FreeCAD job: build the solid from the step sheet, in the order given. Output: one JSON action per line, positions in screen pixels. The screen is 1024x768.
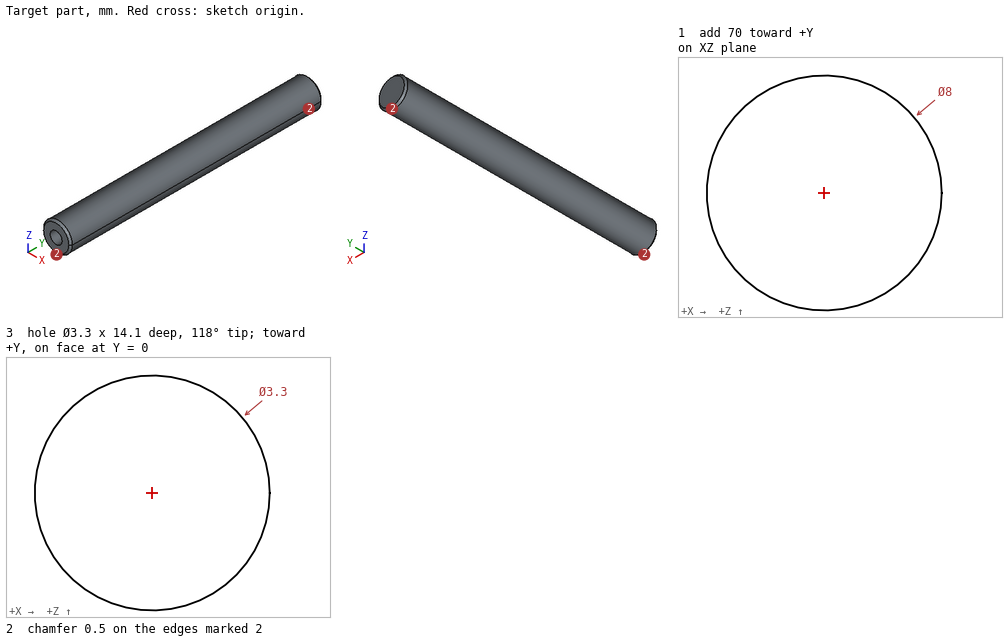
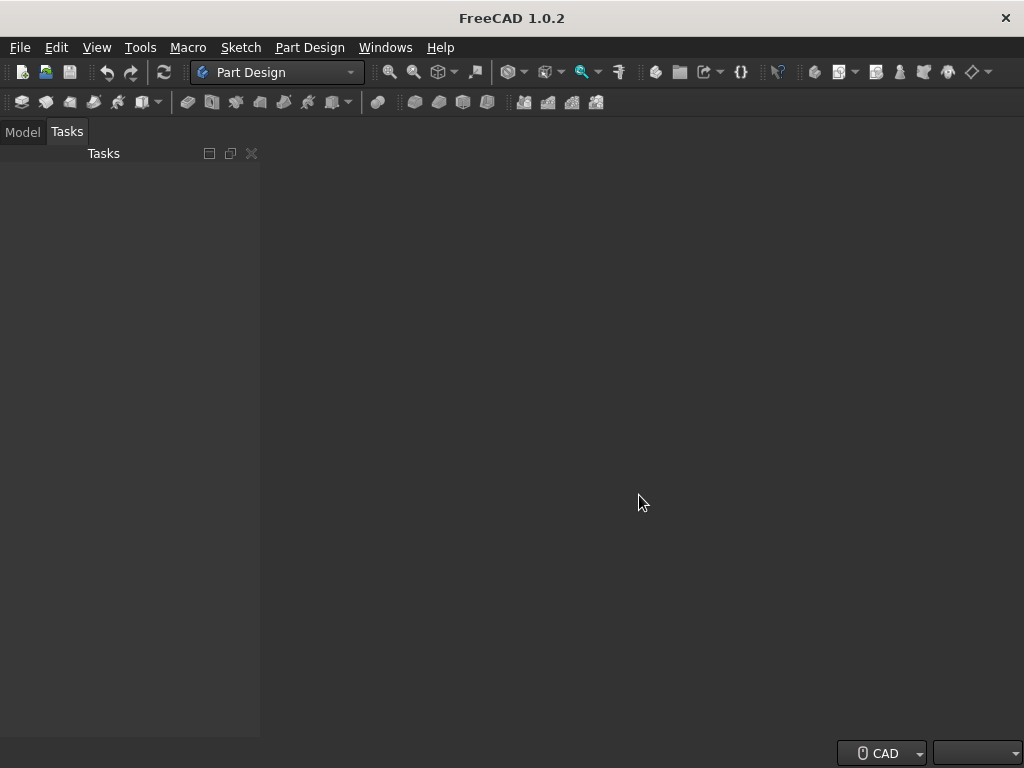
{"action": "key", "text": "ctrl+n"}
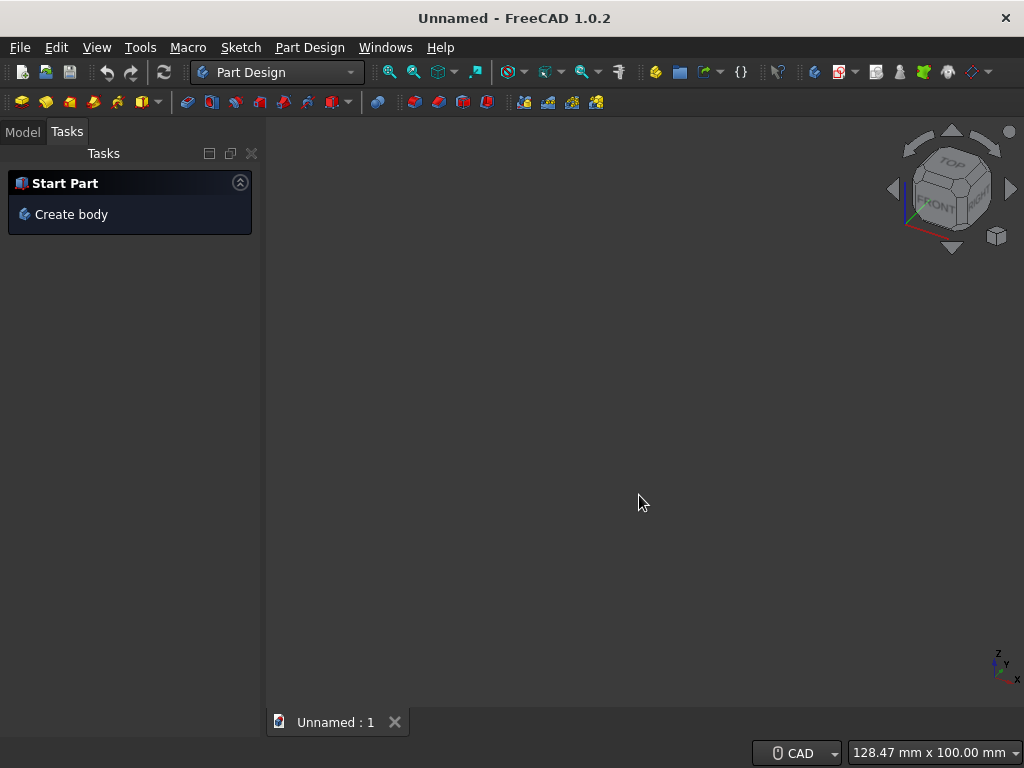
{"action": "left_click", "coordinate": [840, 72]}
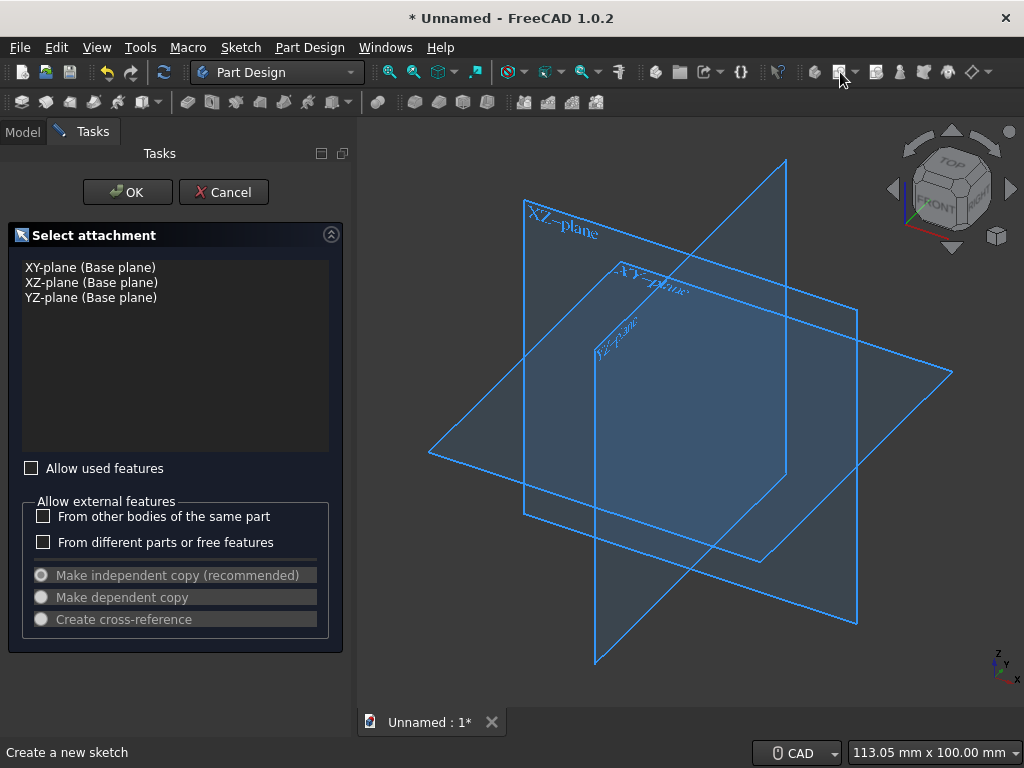
{"action": "left_click", "coordinate": [82, 282]}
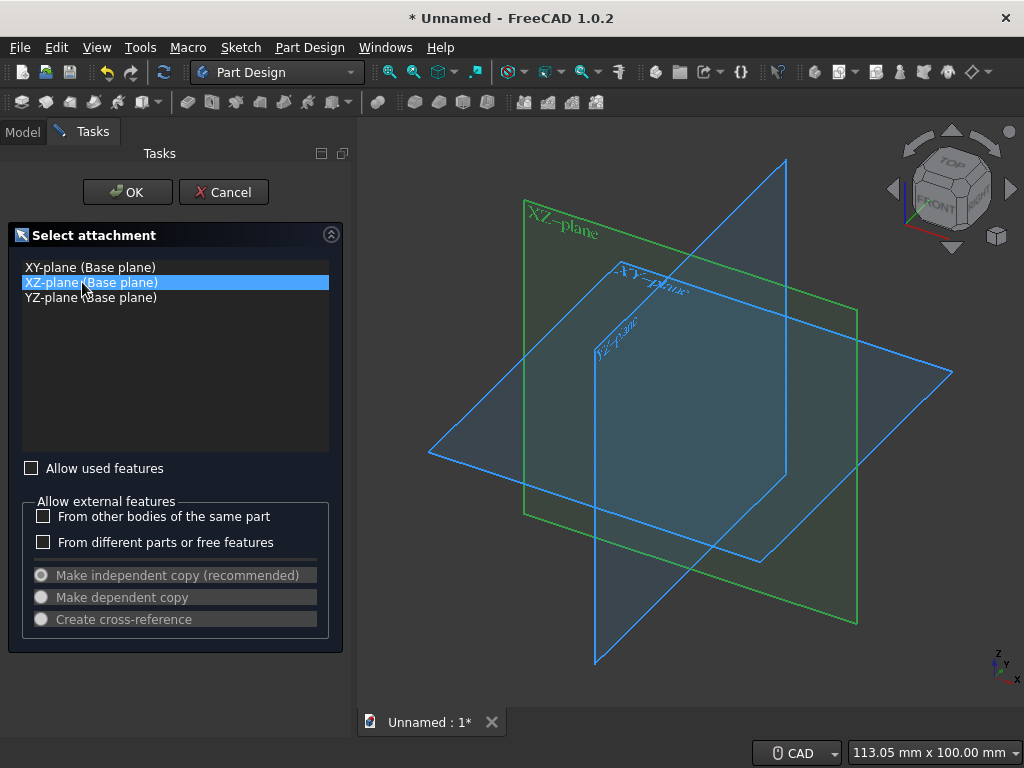
{"action": "left_click", "coordinate": [128, 192]}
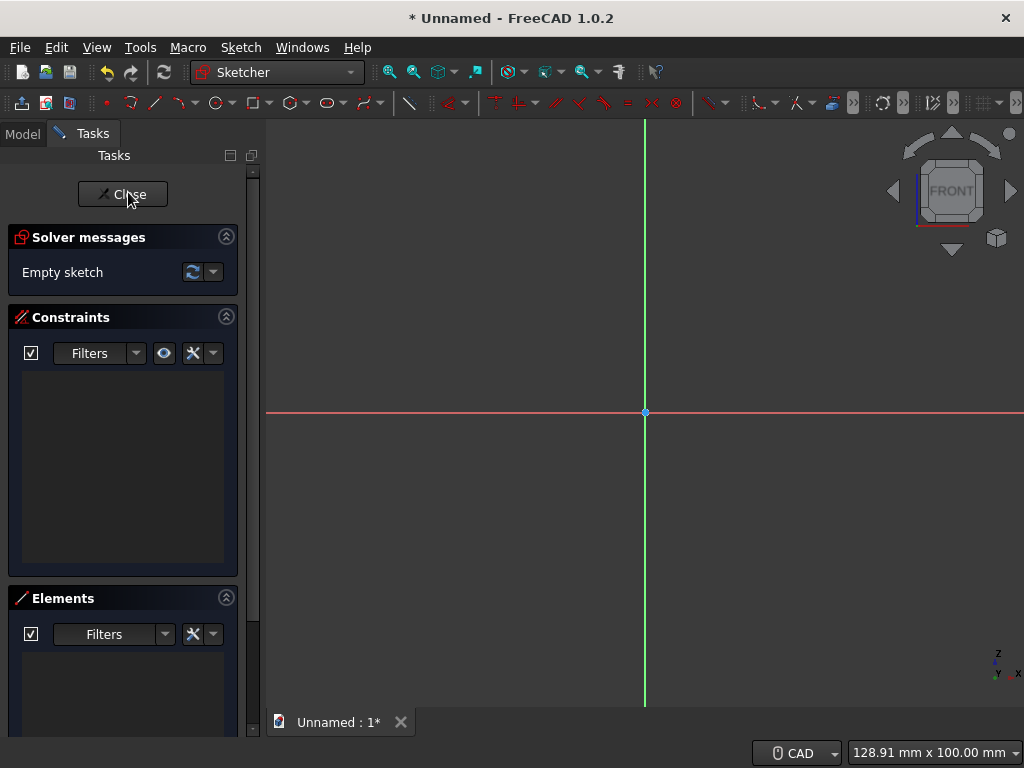
{"action": "scroll", "coordinate": [656, 413], "scroll_direction": "up", "scroll_amount": 10}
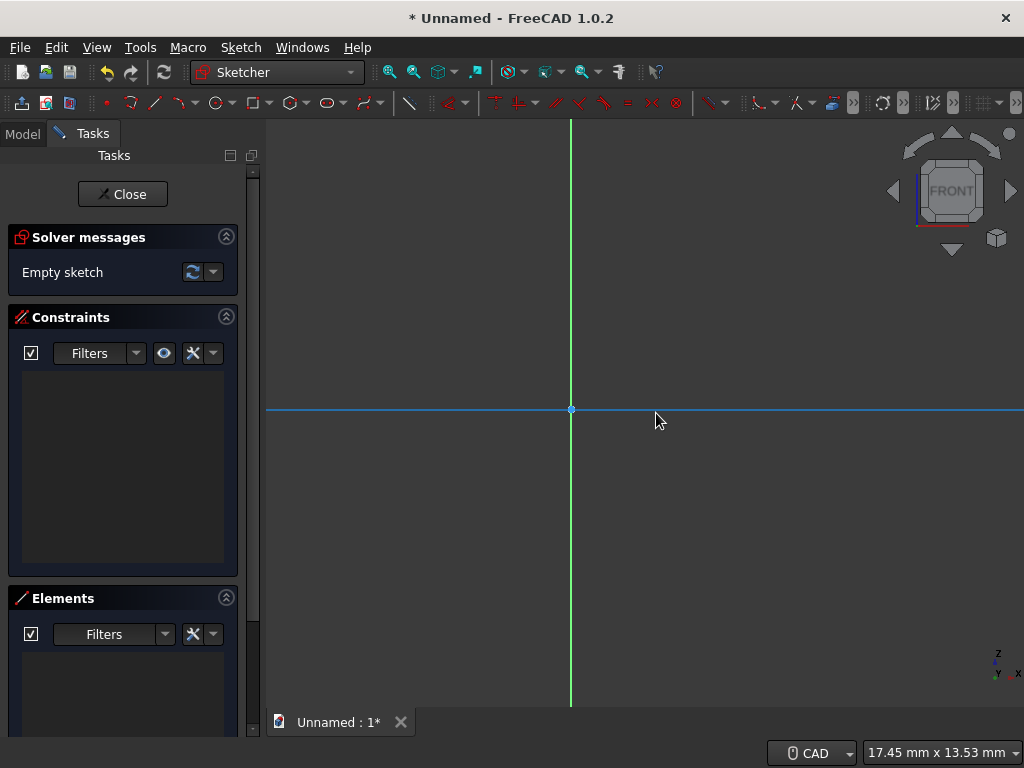
{"action": "key", "text": "g c"}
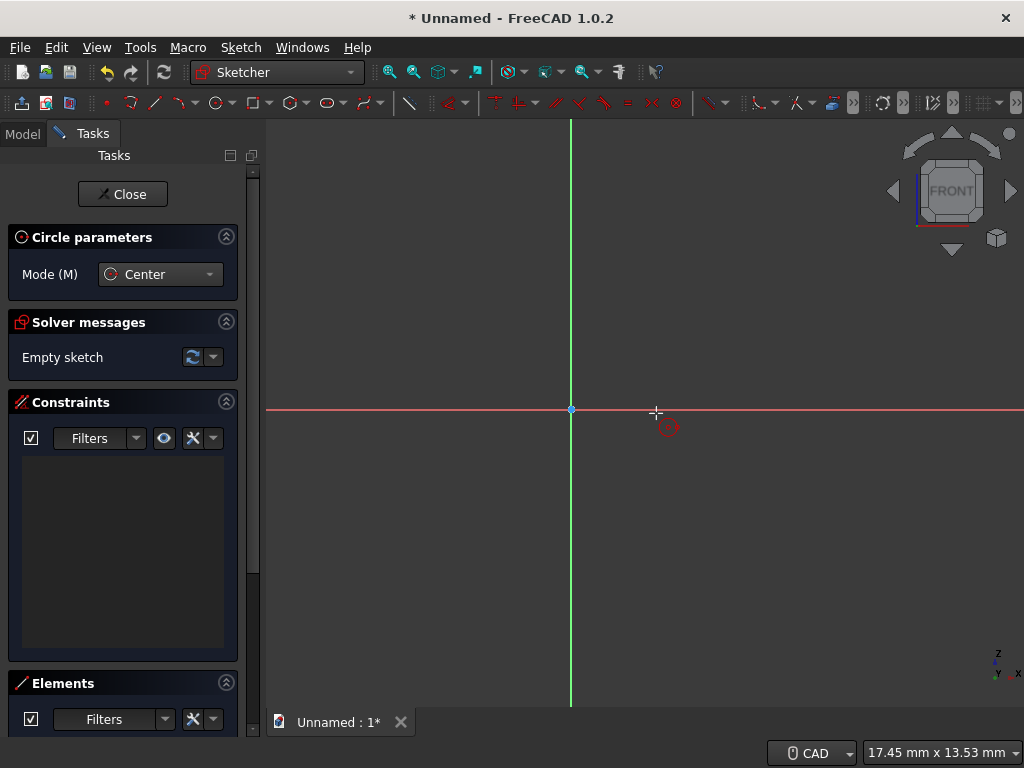
{"action": "left_click", "coordinate": [571, 410]}
{"action": "left_click", "coordinate": [694, 287]}
{"action": "key", "text": "Escape"}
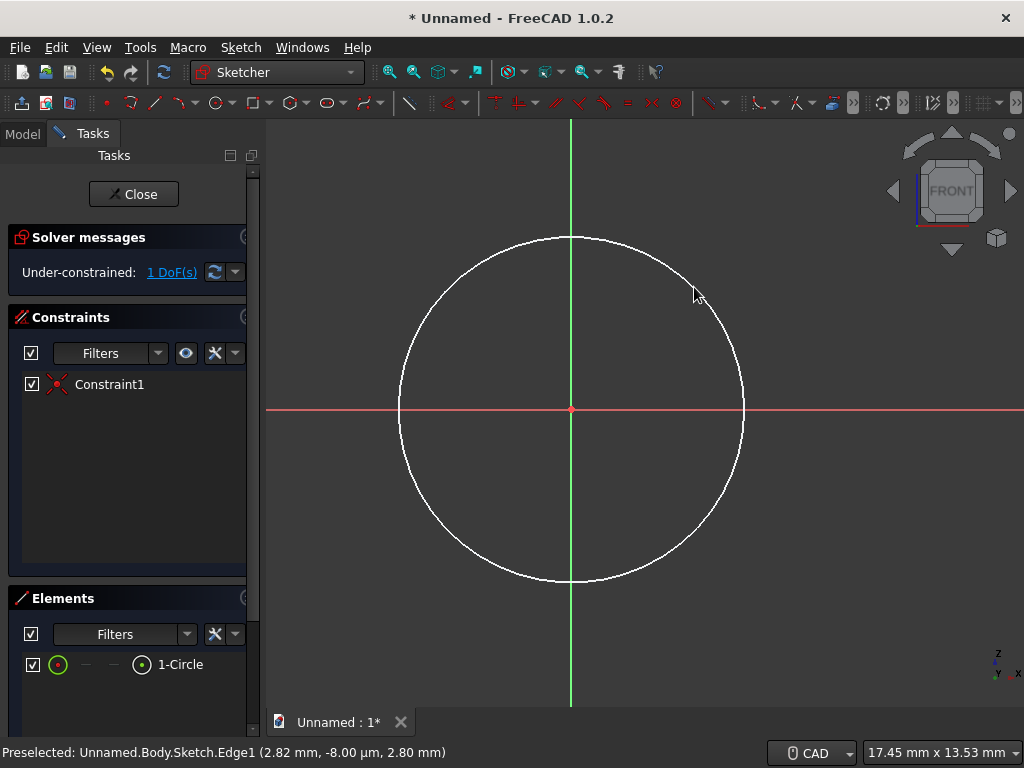
{"action": "left_click", "coordinate": [693, 287]}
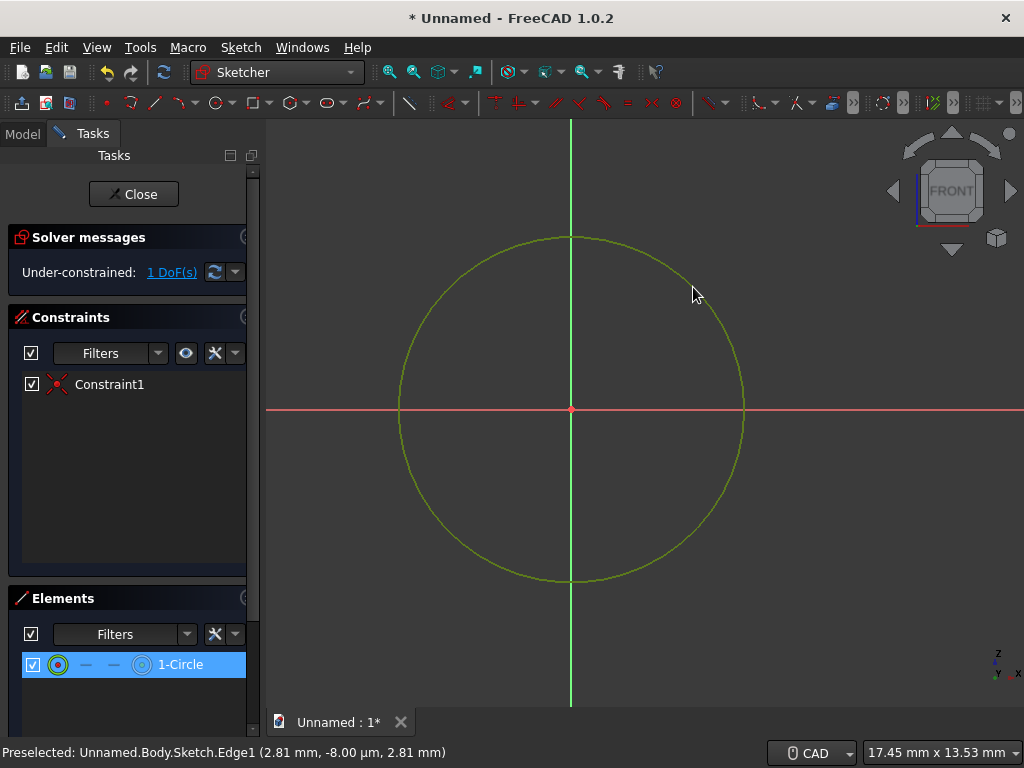
{"action": "left_click", "coordinate": [468, 104]}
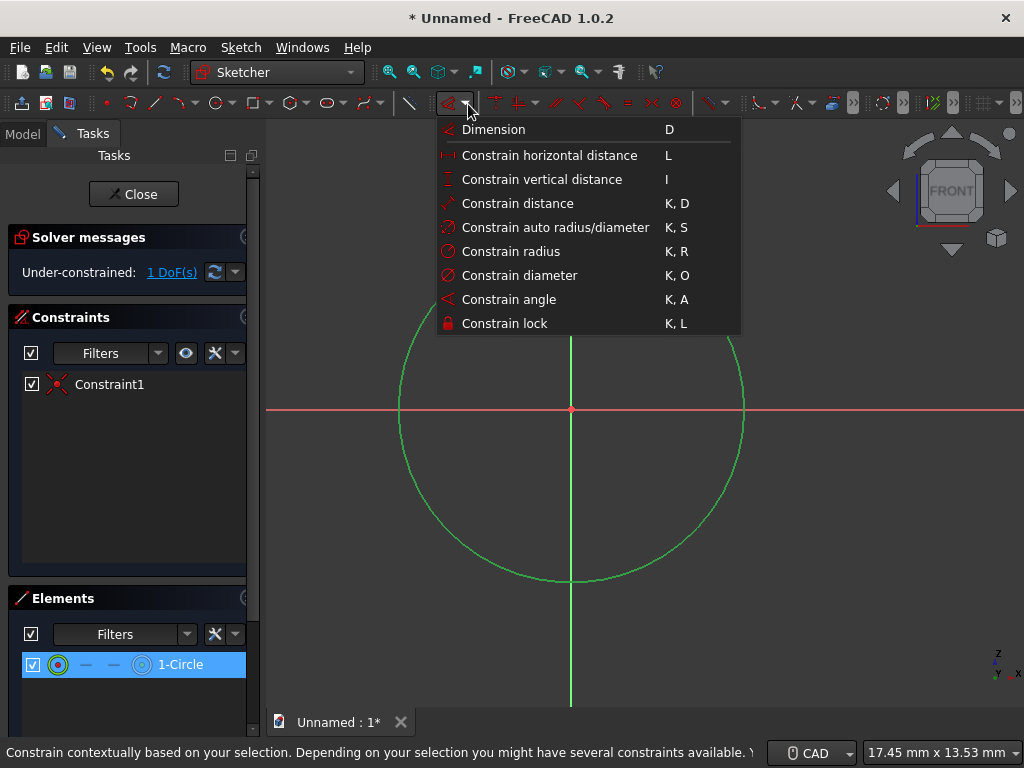
{"action": "left_click", "coordinate": [589, 275]}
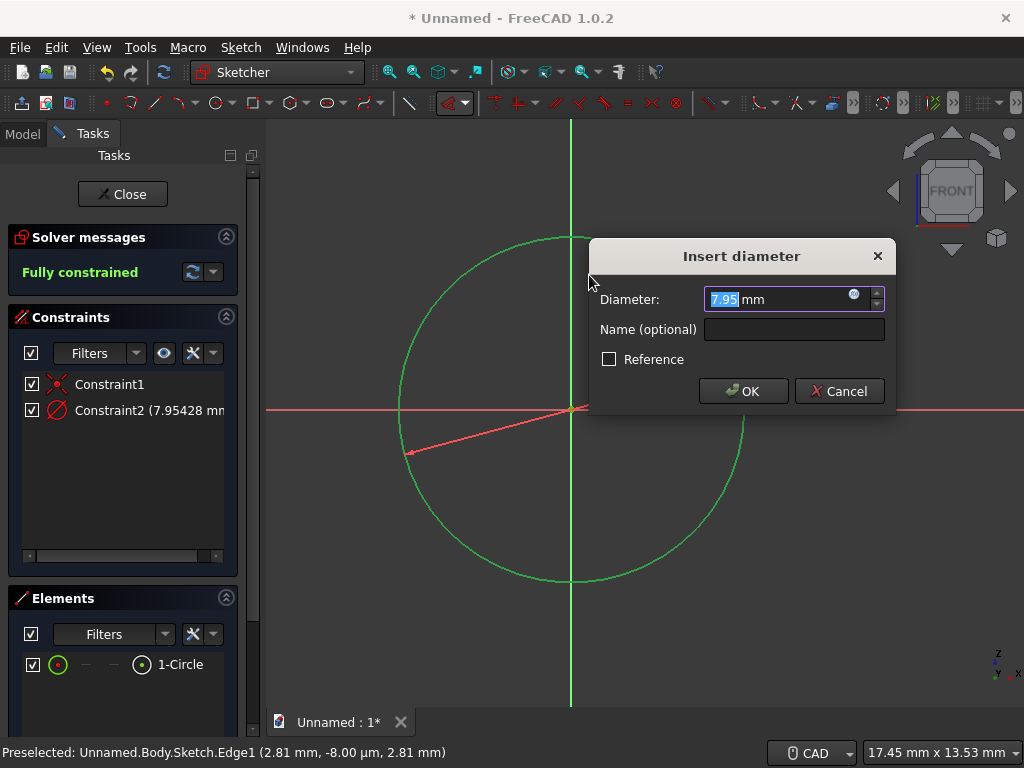
{"action": "type", "text": "8"}
{"action": "key", "text": "Return"}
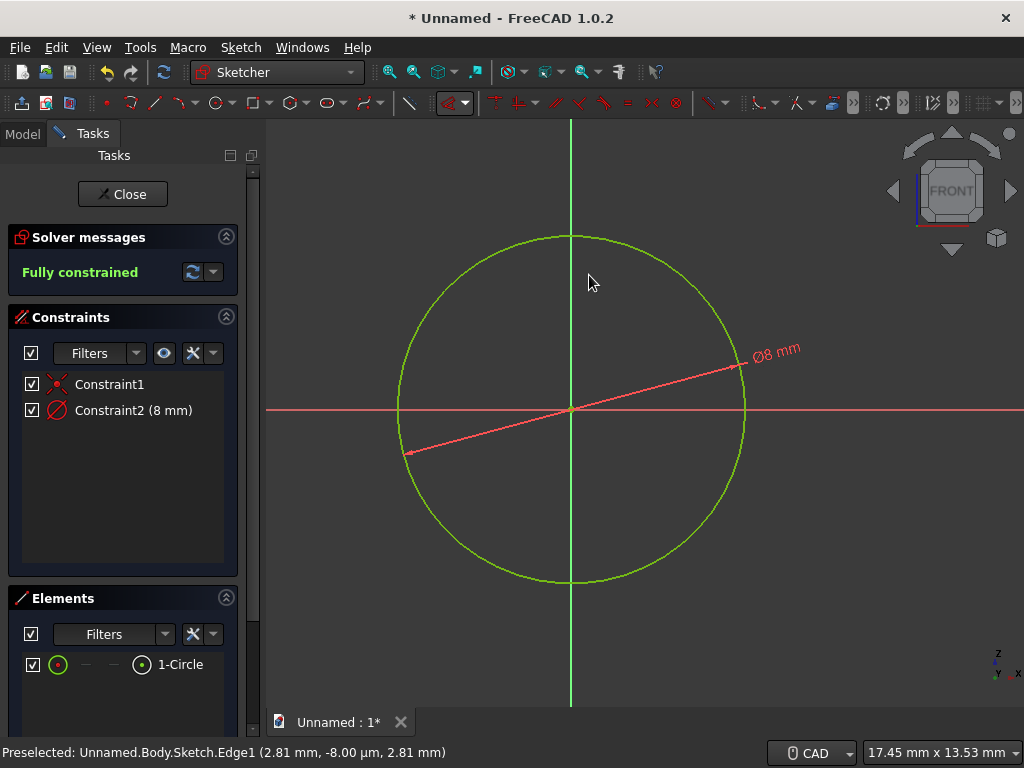
{"action": "left_click", "coordinate": [123, 194]}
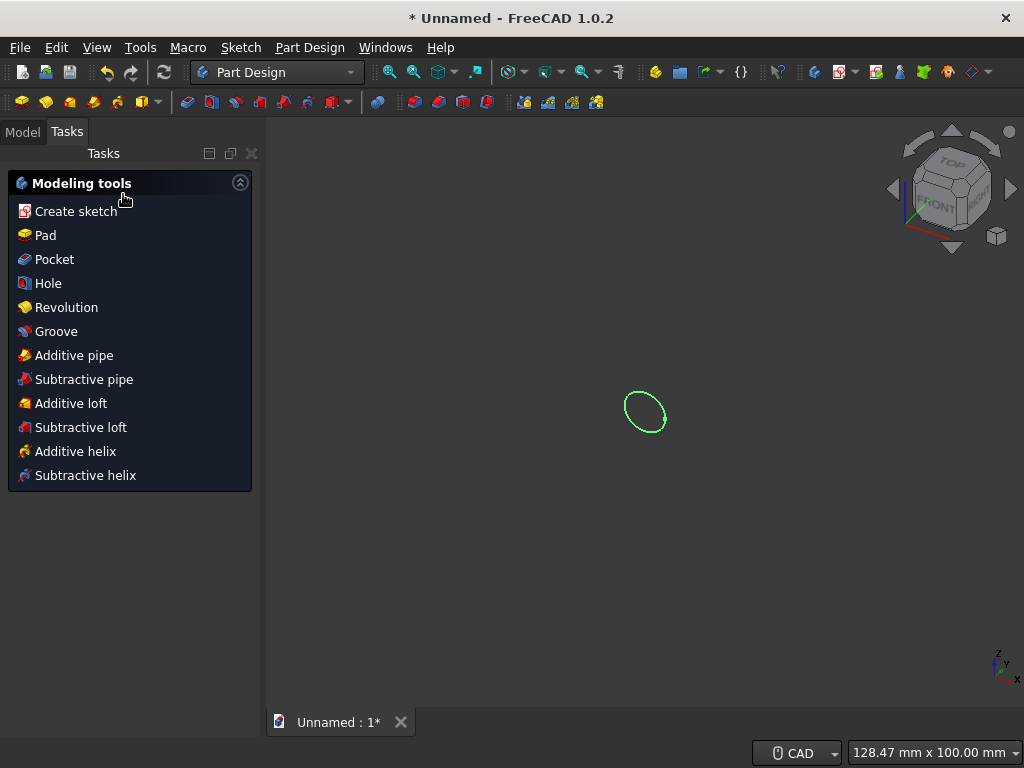
{"action": "left_click", "coordinate": [22, 102]}